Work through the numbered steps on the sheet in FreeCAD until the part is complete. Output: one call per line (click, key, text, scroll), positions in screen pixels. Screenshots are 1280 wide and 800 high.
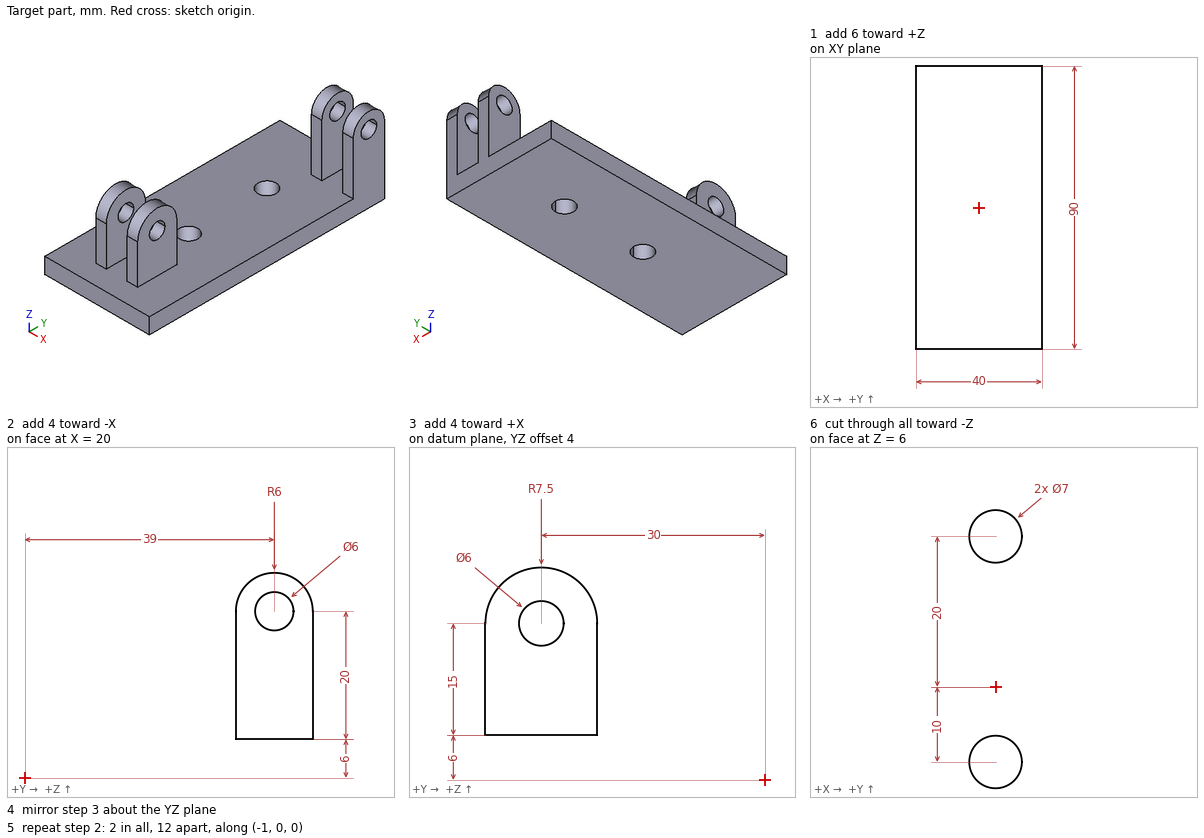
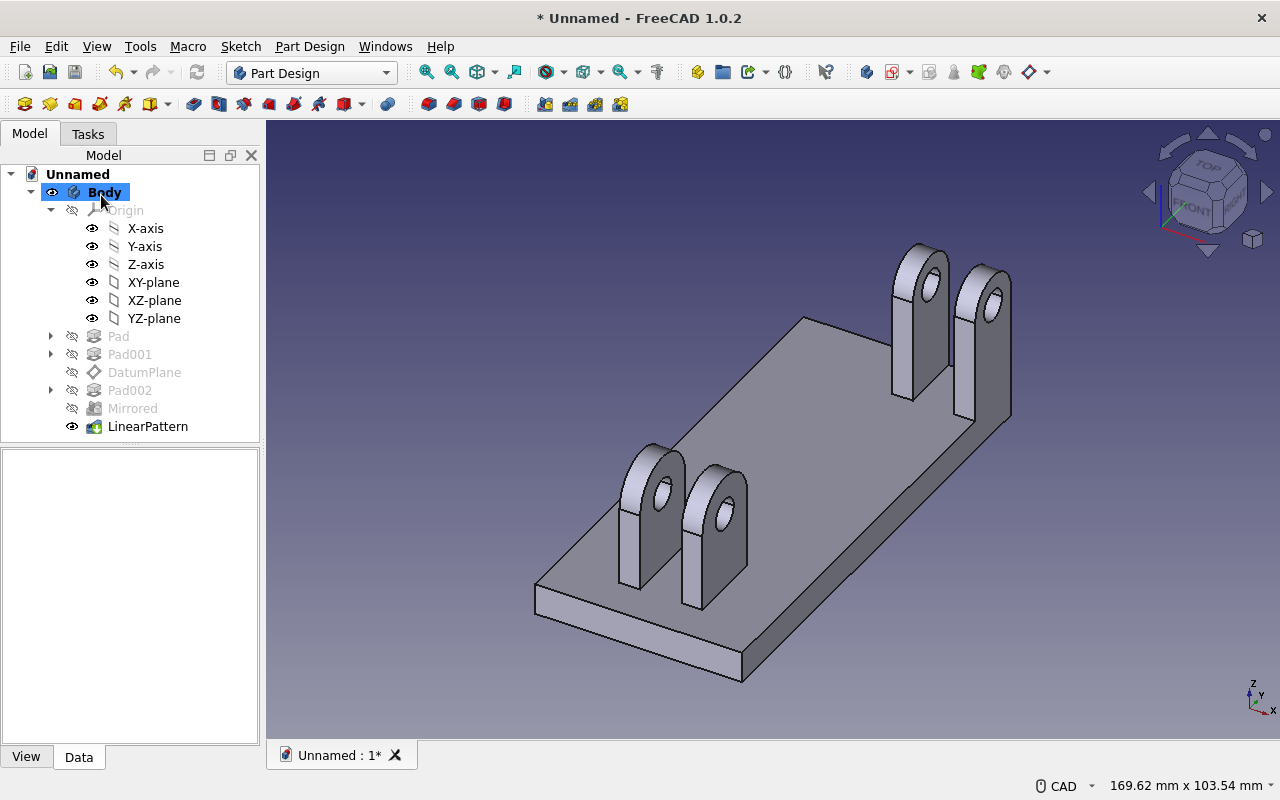
click(811, 446)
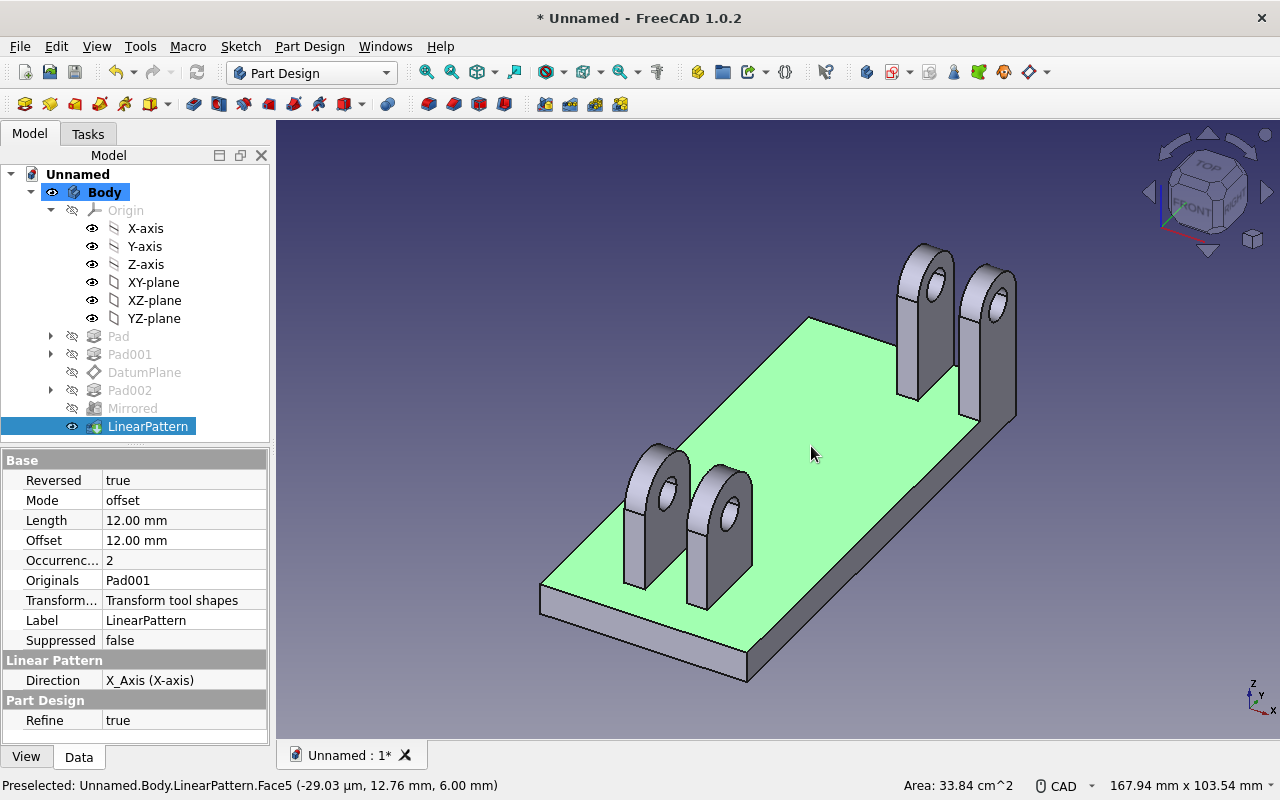
click(892, 72)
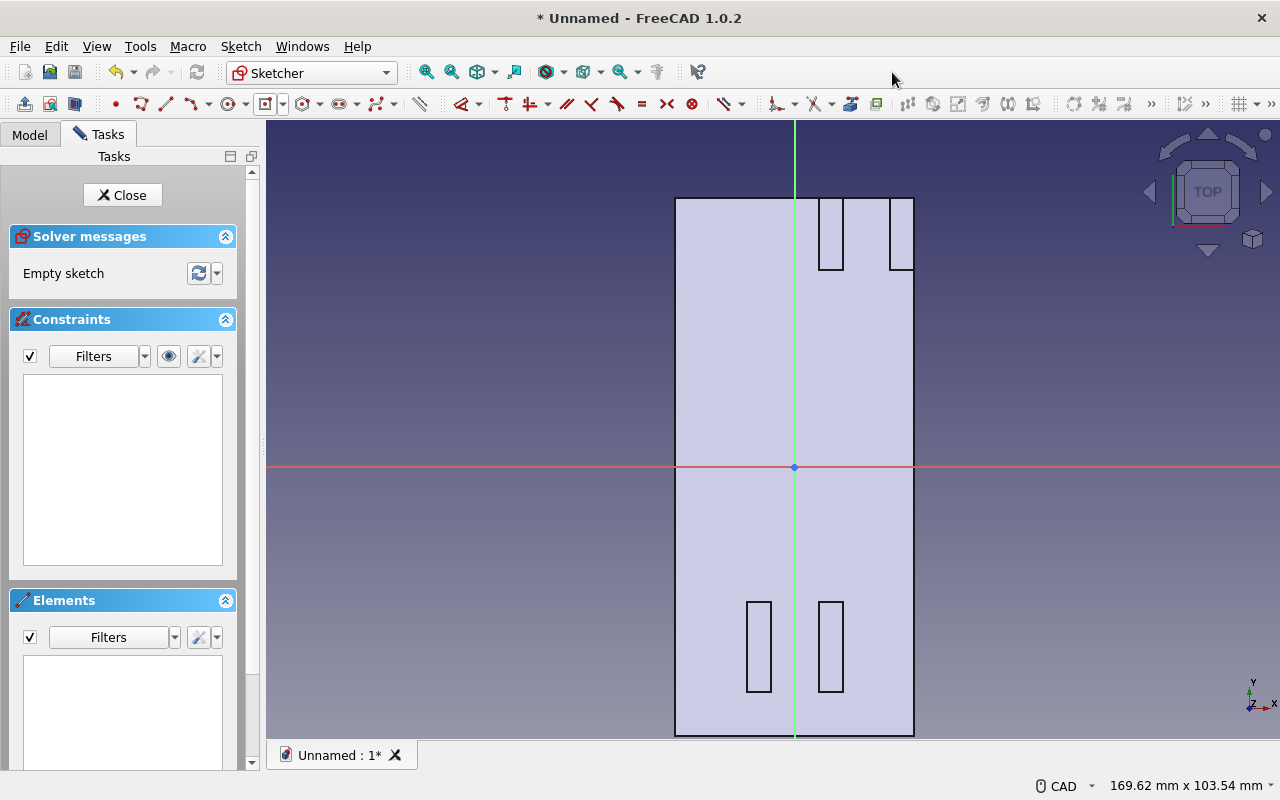
scroll(905, 447, up, 3)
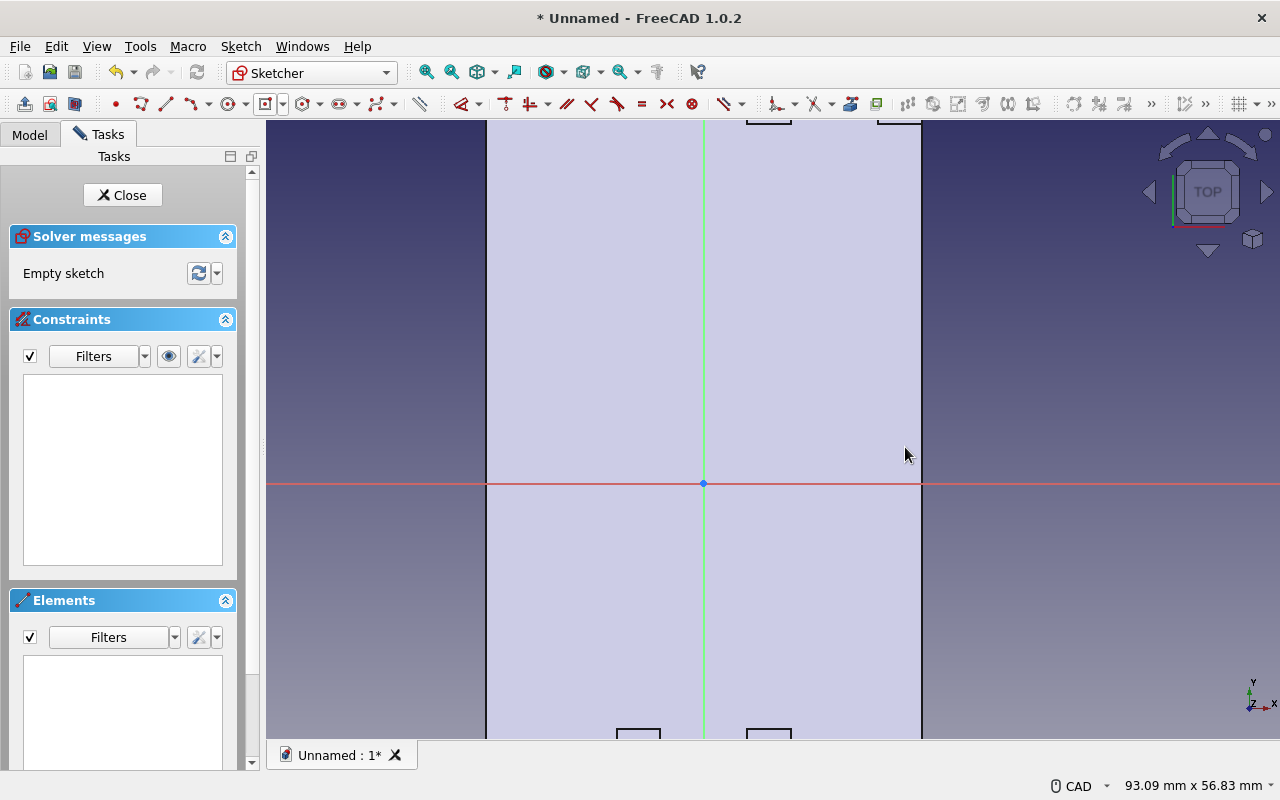
click(228, 104)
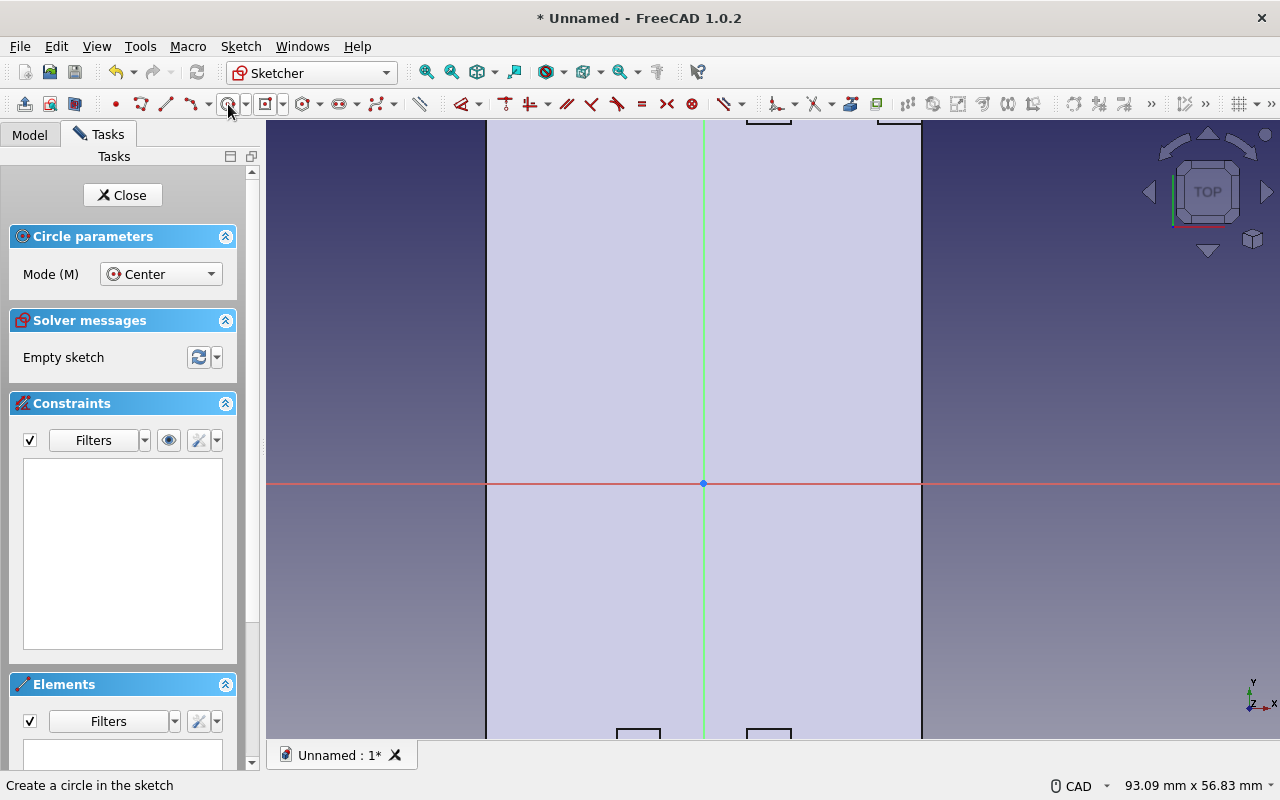
click(704, 266)
move(731, 239)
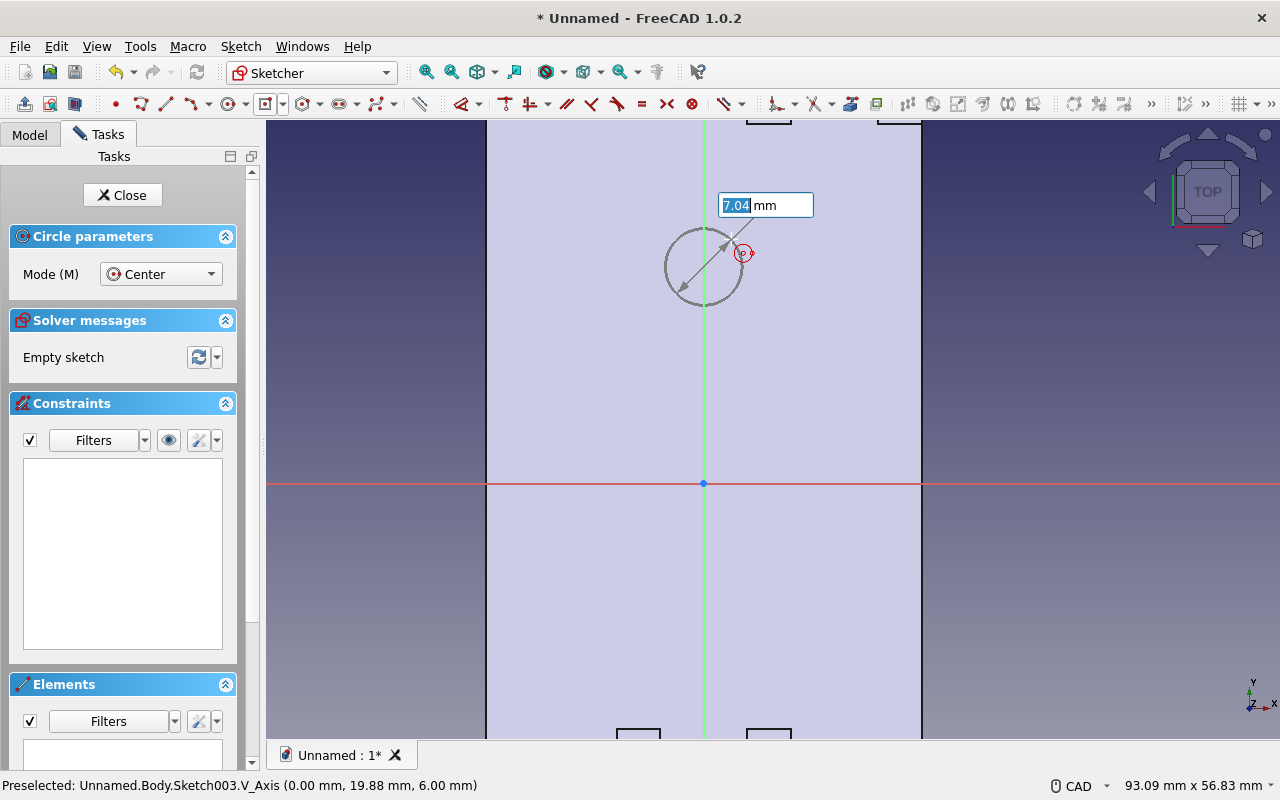
text(7)
key(Return)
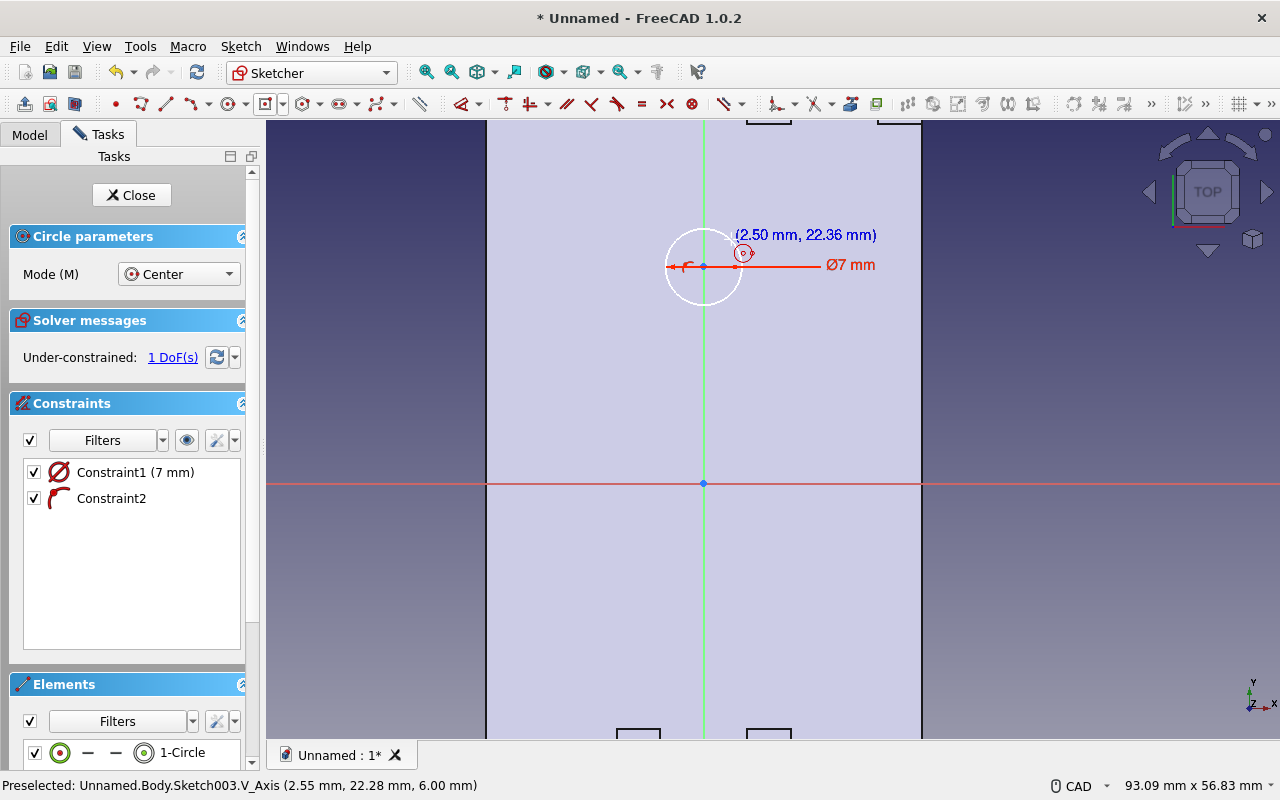
click(704, 593)
move(731, 566)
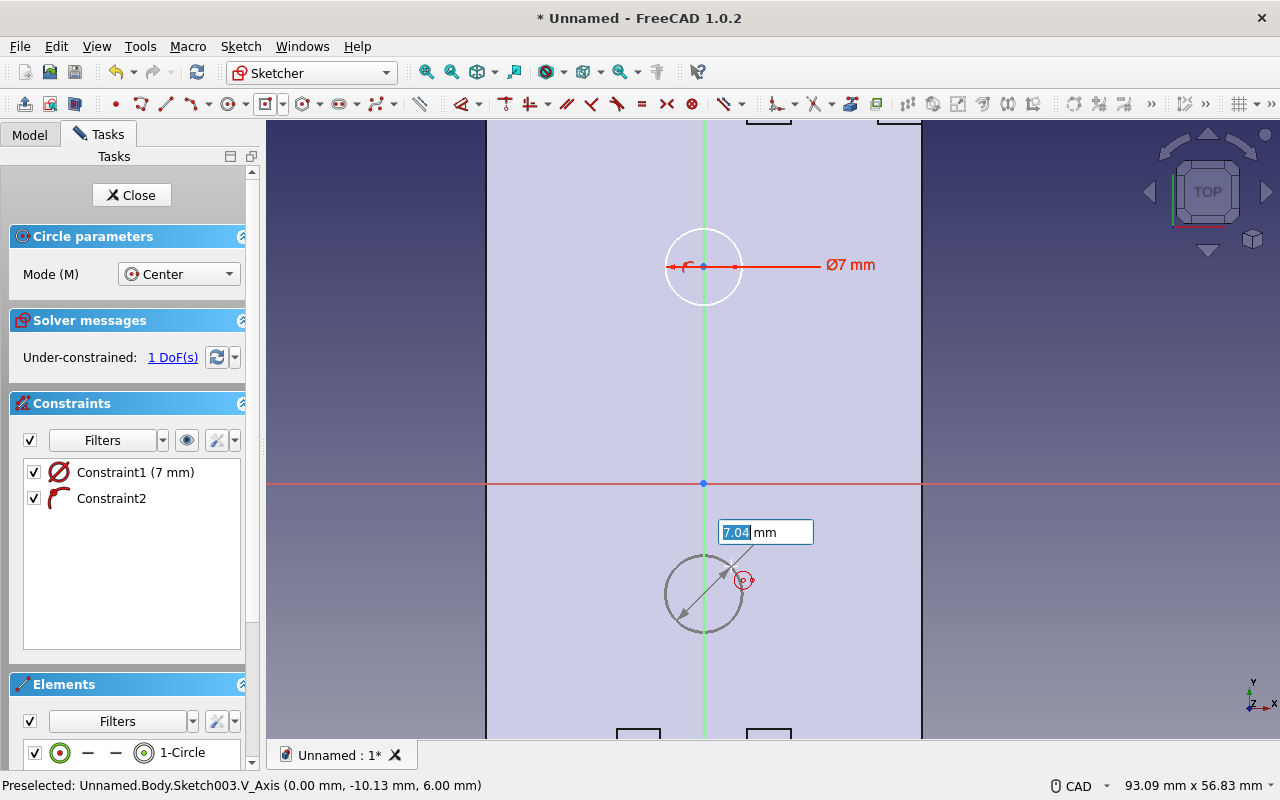
text(7)
key(Return)
key(Escape)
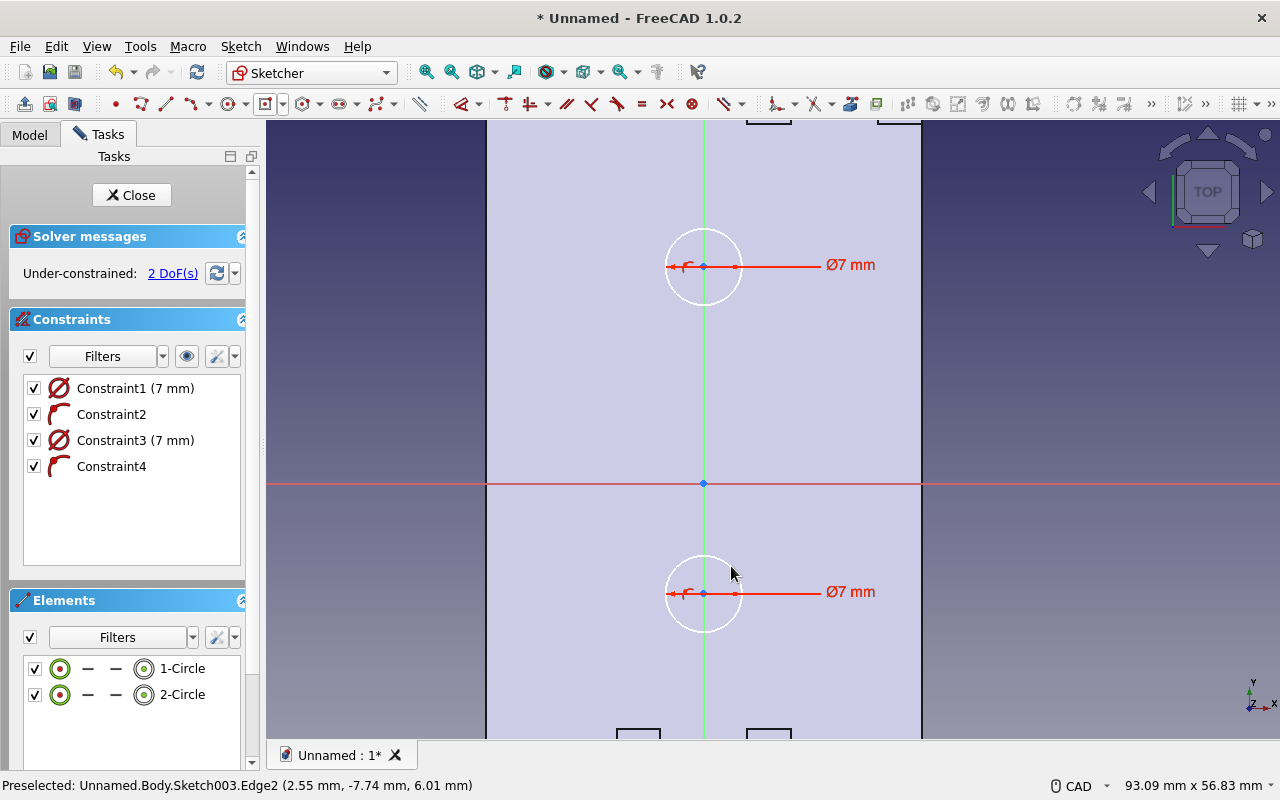
click(460, 104)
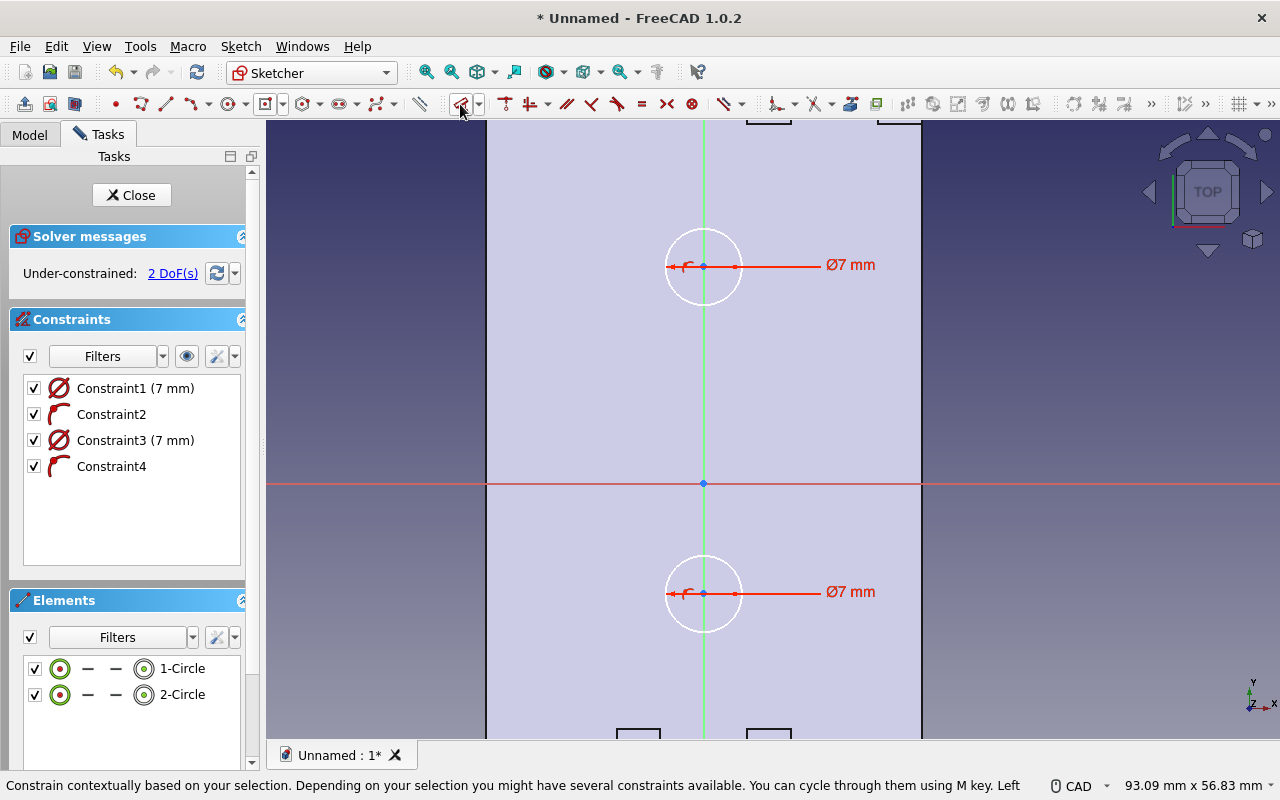
click(704, 267)
click(738, 375)